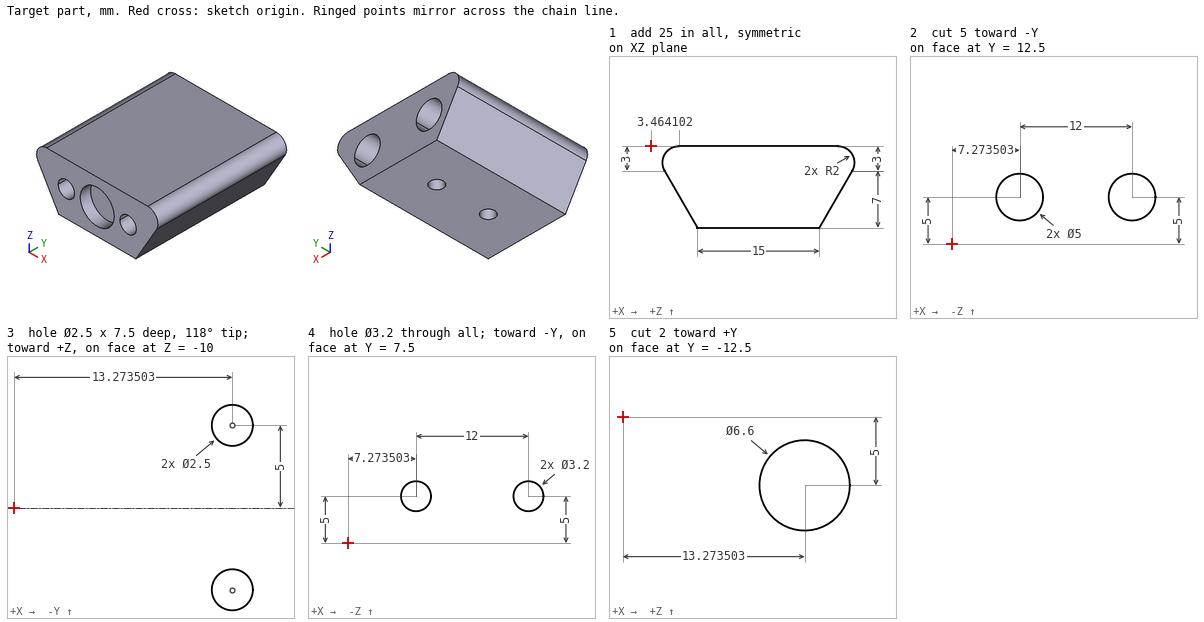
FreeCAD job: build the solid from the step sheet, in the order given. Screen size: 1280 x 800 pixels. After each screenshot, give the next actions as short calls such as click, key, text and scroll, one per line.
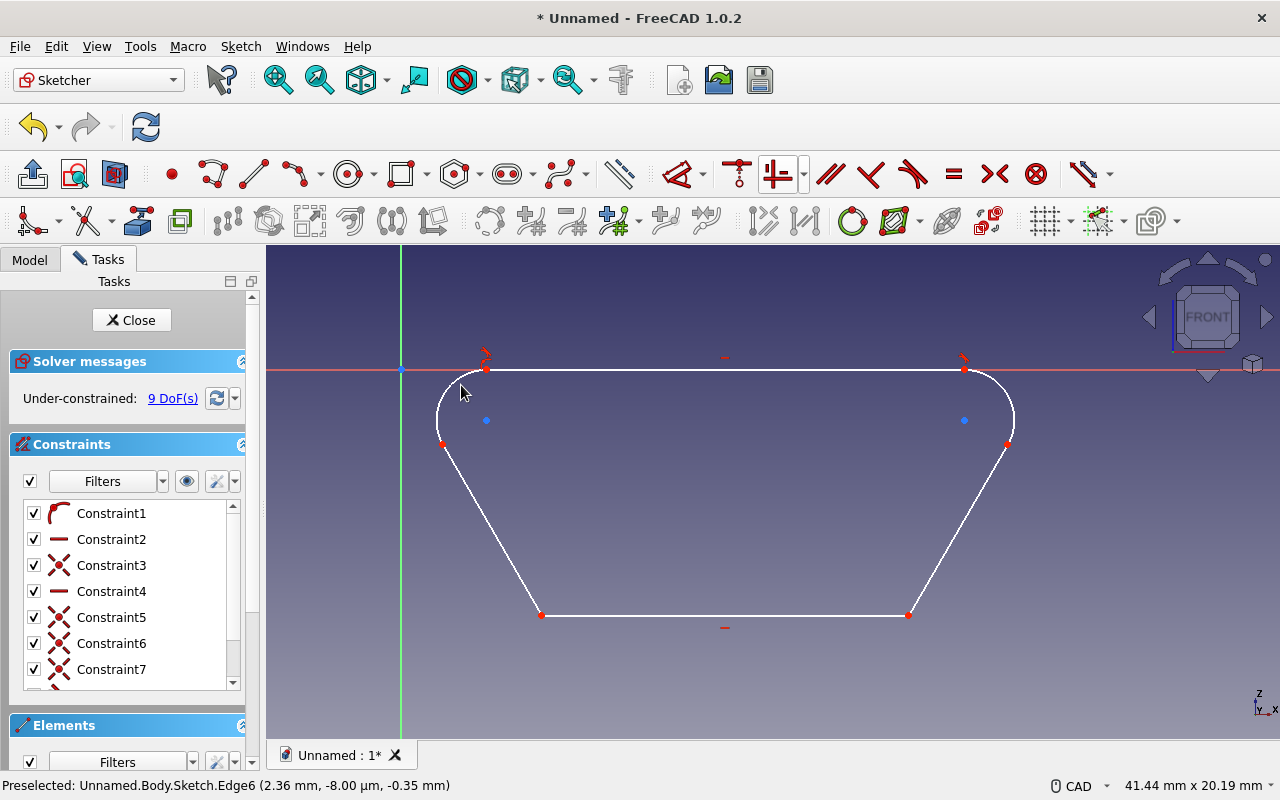
click(978, 496)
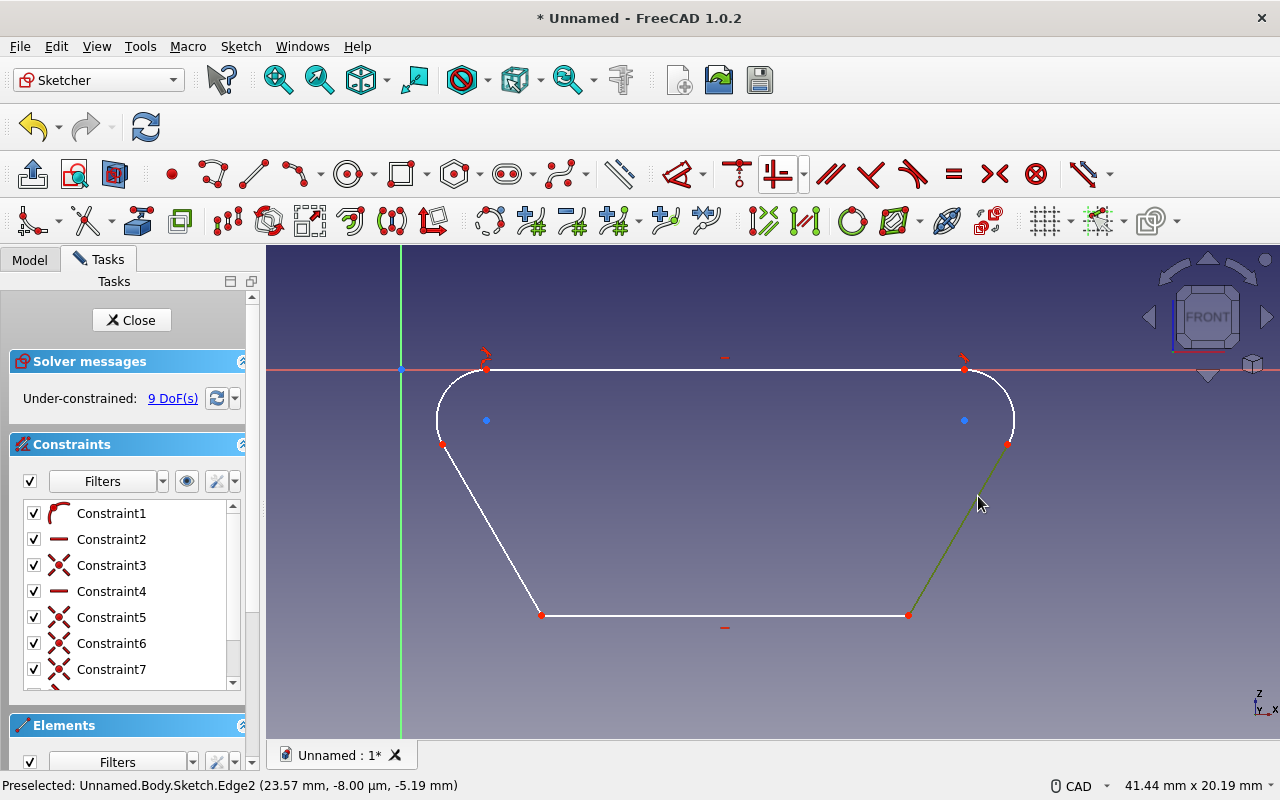
click(1014, 414)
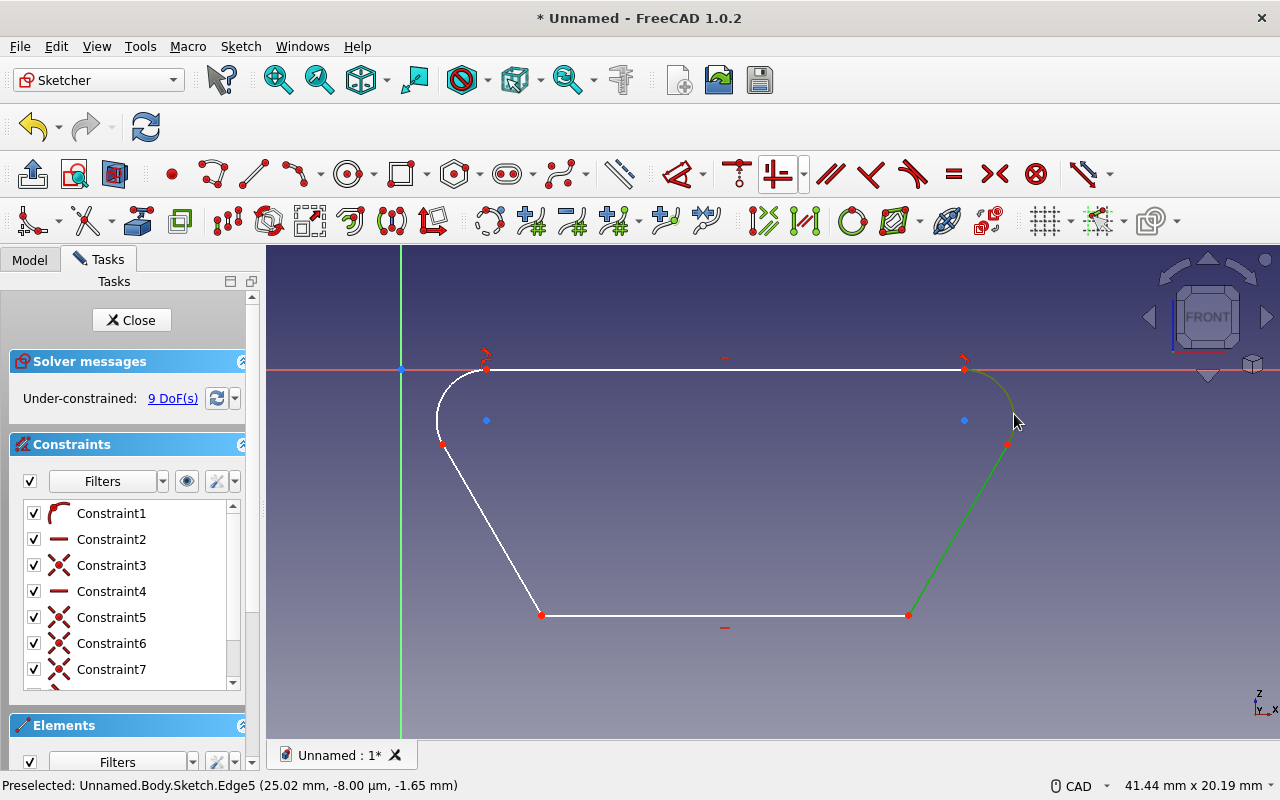
click(913, 174)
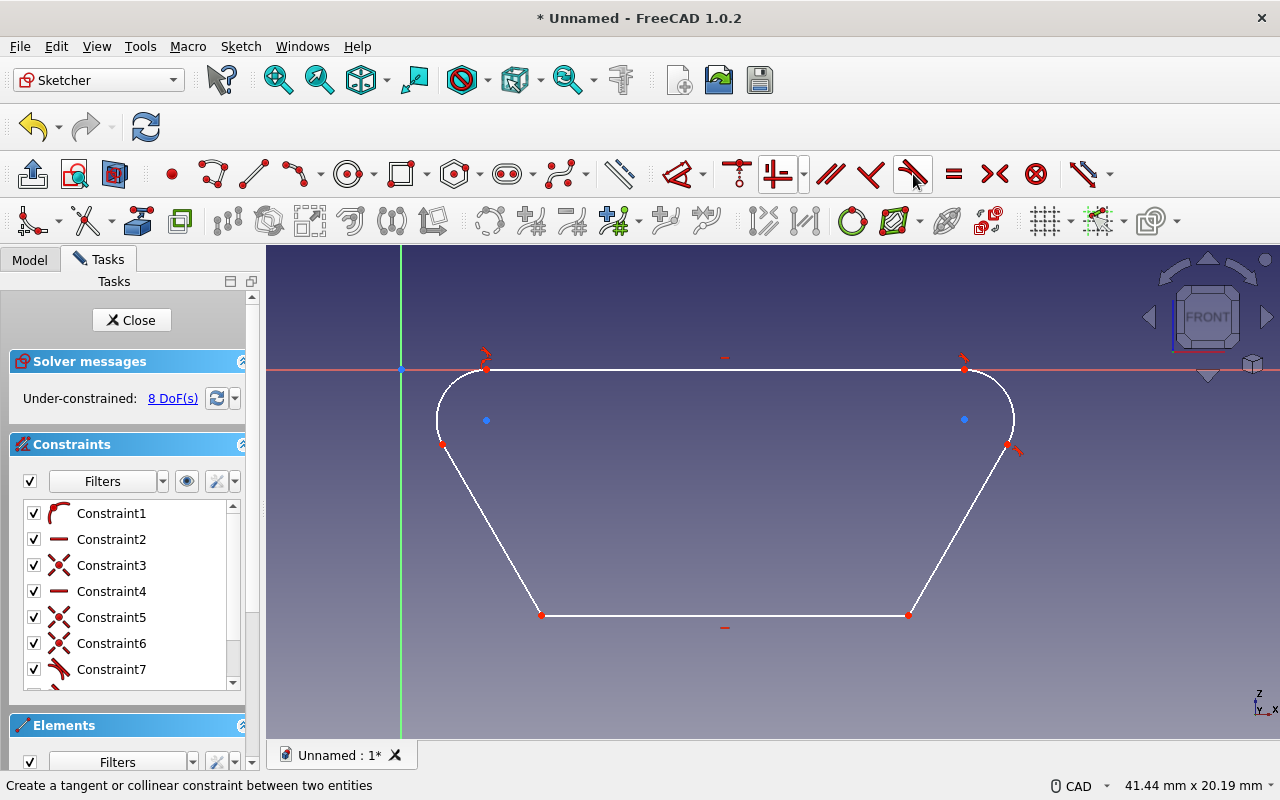
click(512, 564)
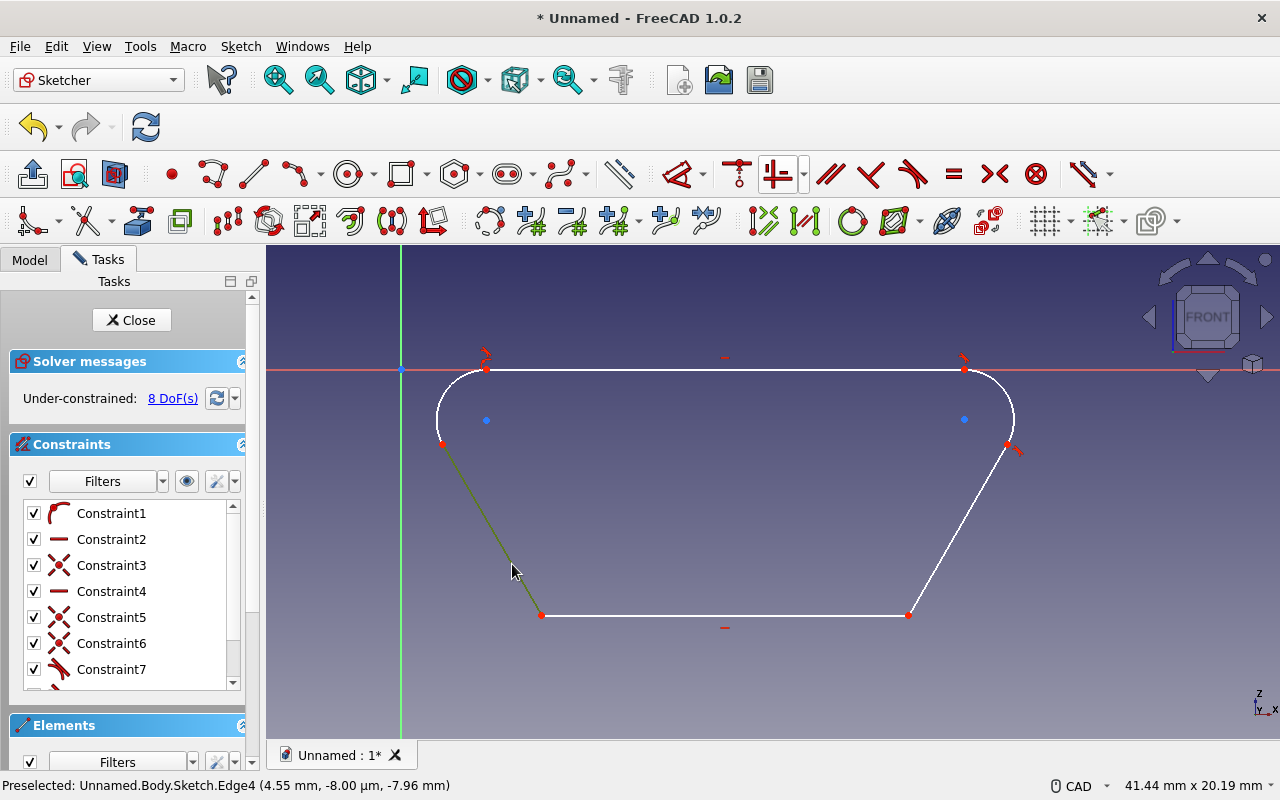
scroll(458, 379, up, 2)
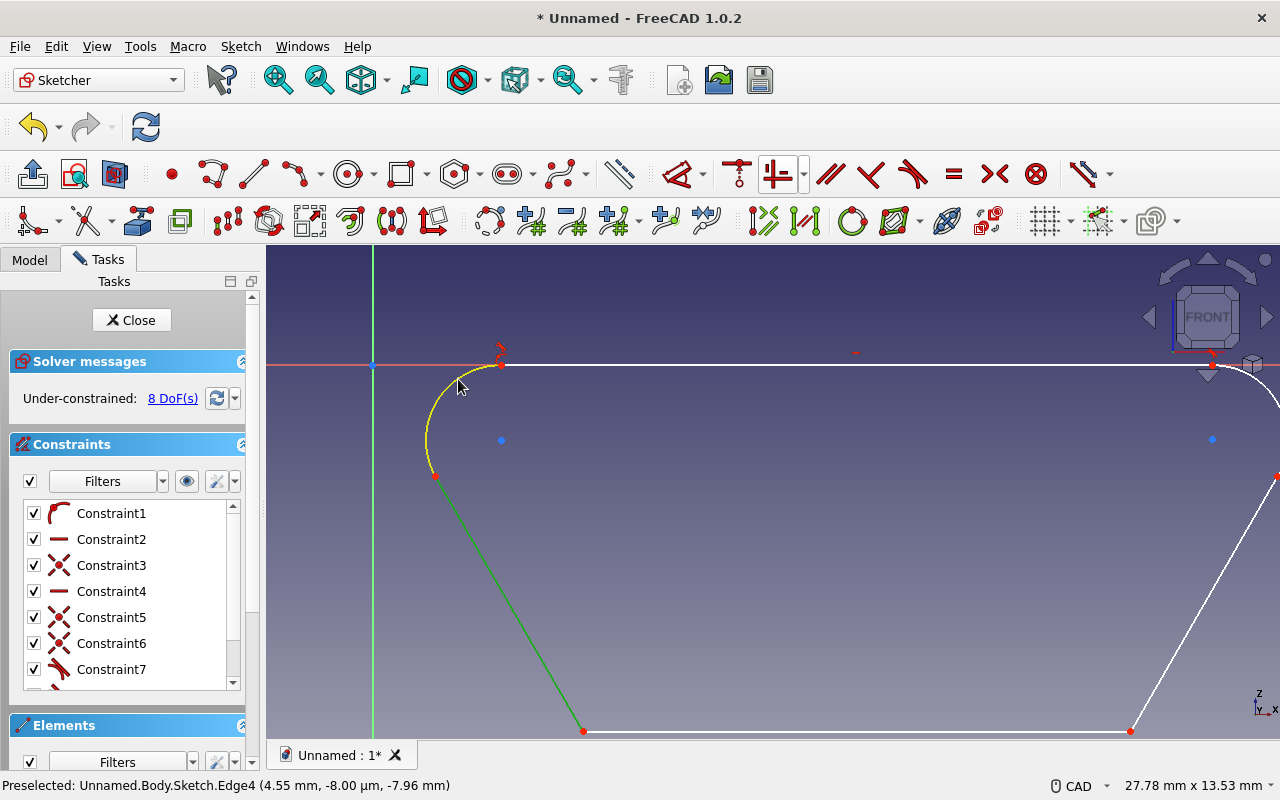
click(457, 379)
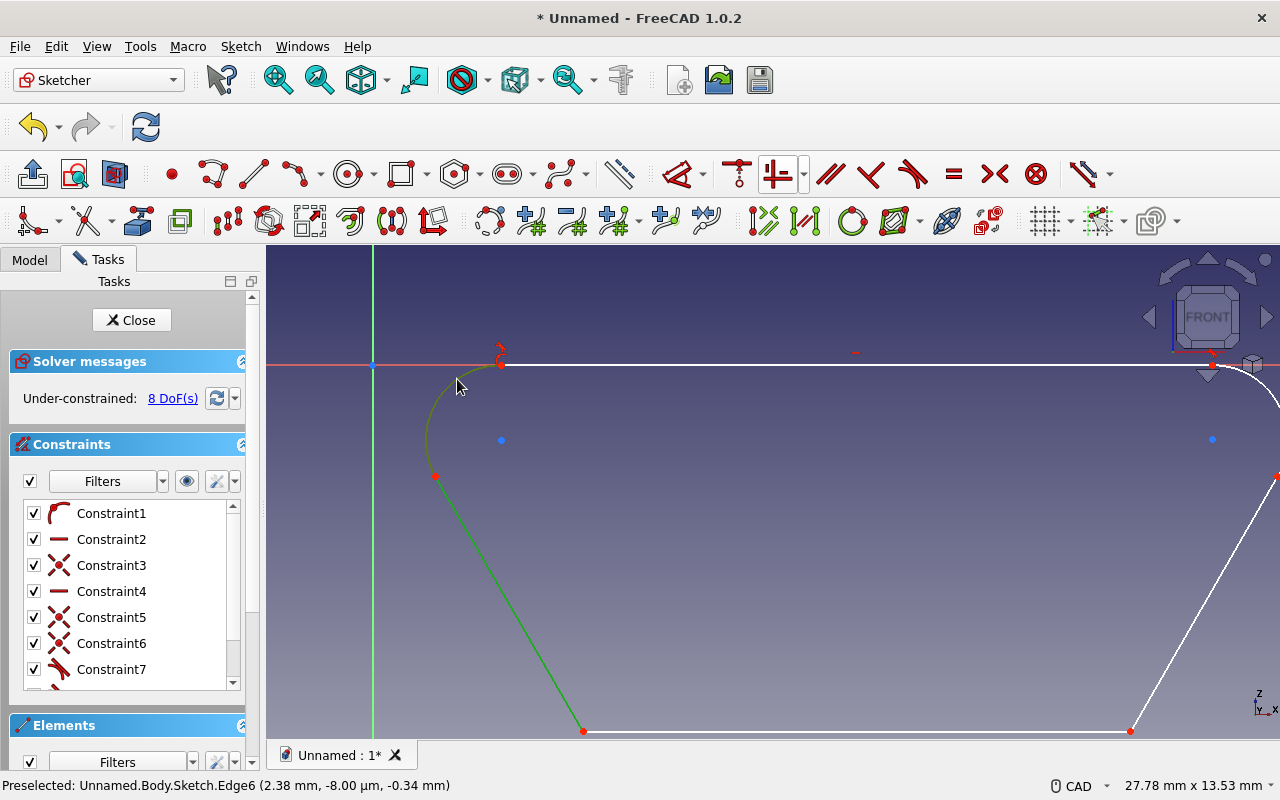
click(913, 174)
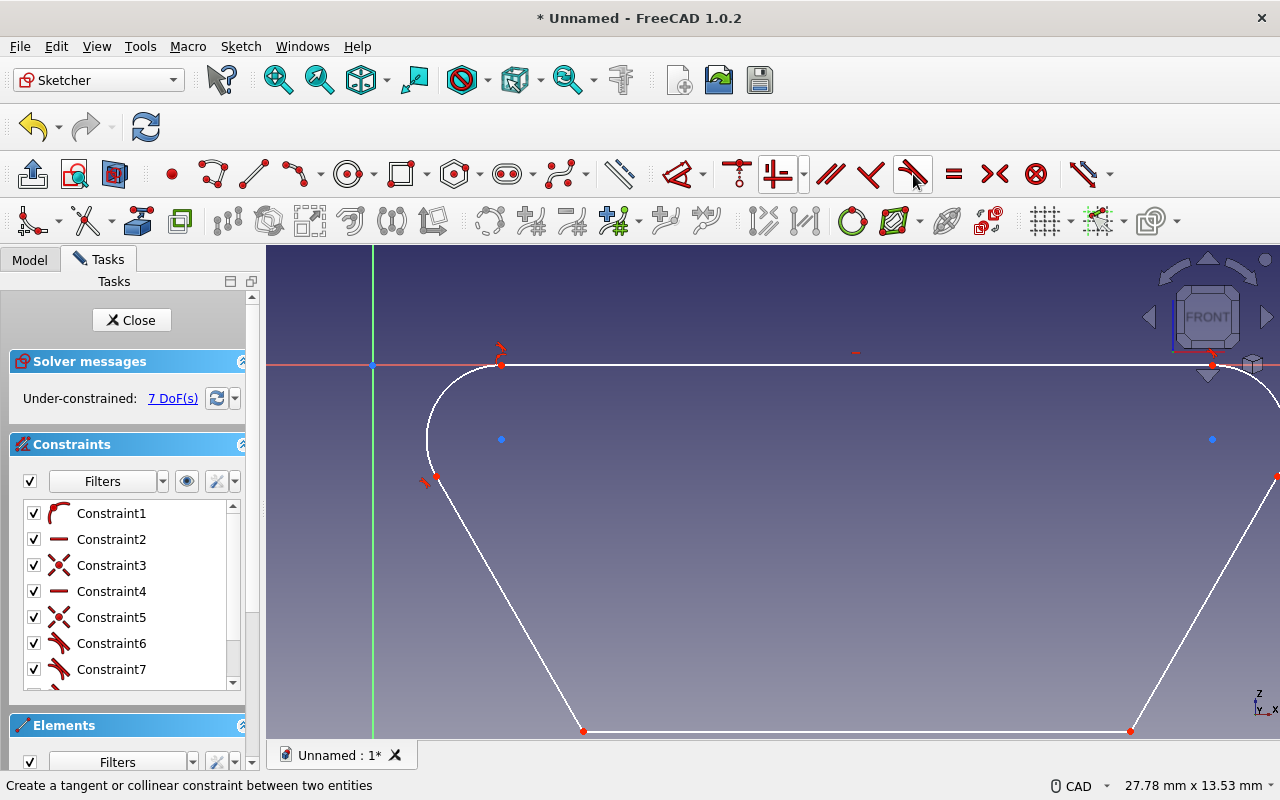
scroll(458, 379, down, 2)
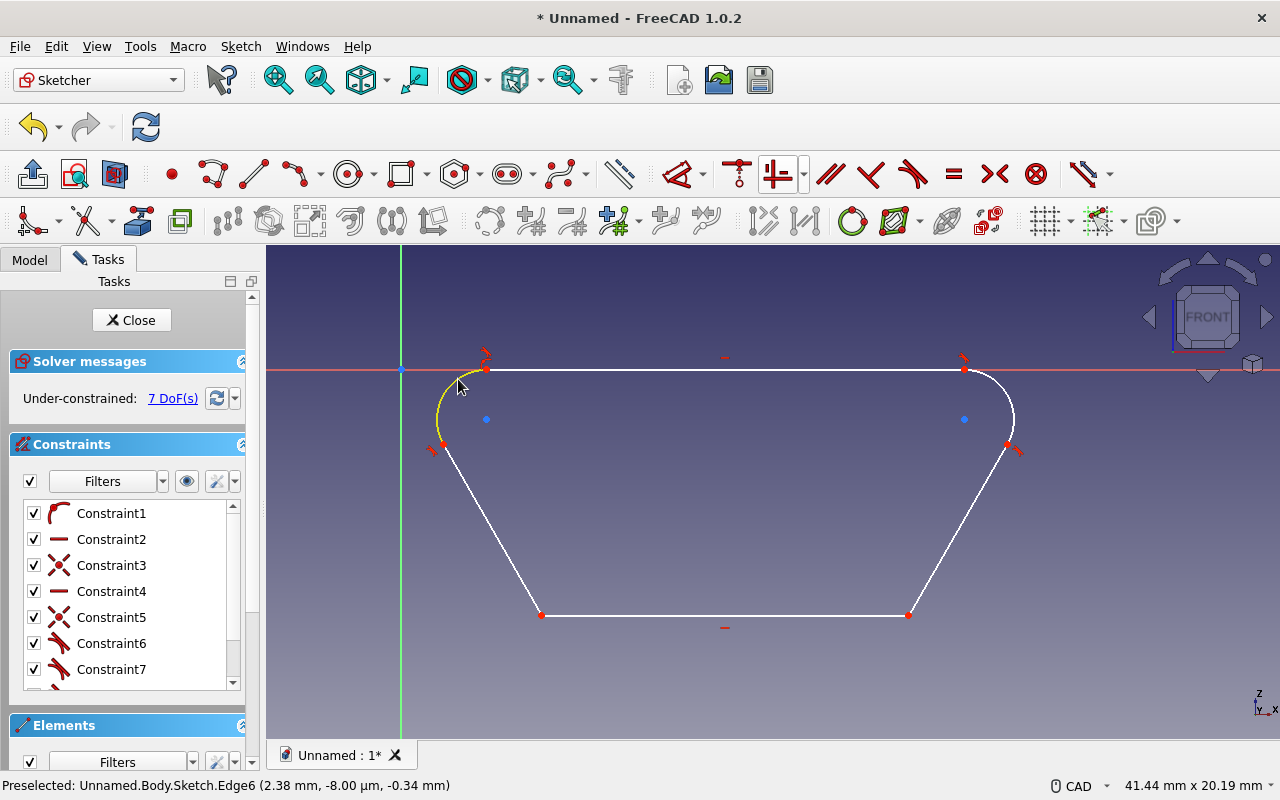
click(1014, 414)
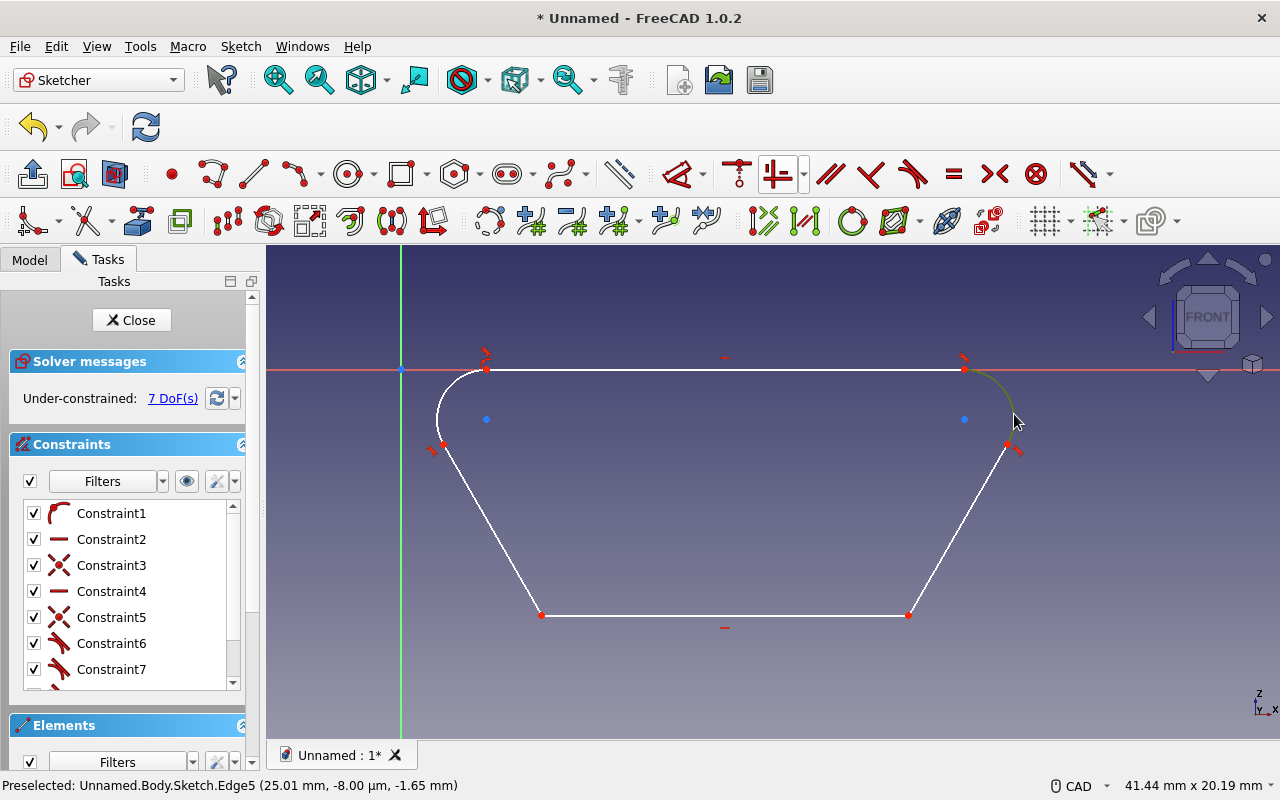
scroll(458, 379, up, 2)